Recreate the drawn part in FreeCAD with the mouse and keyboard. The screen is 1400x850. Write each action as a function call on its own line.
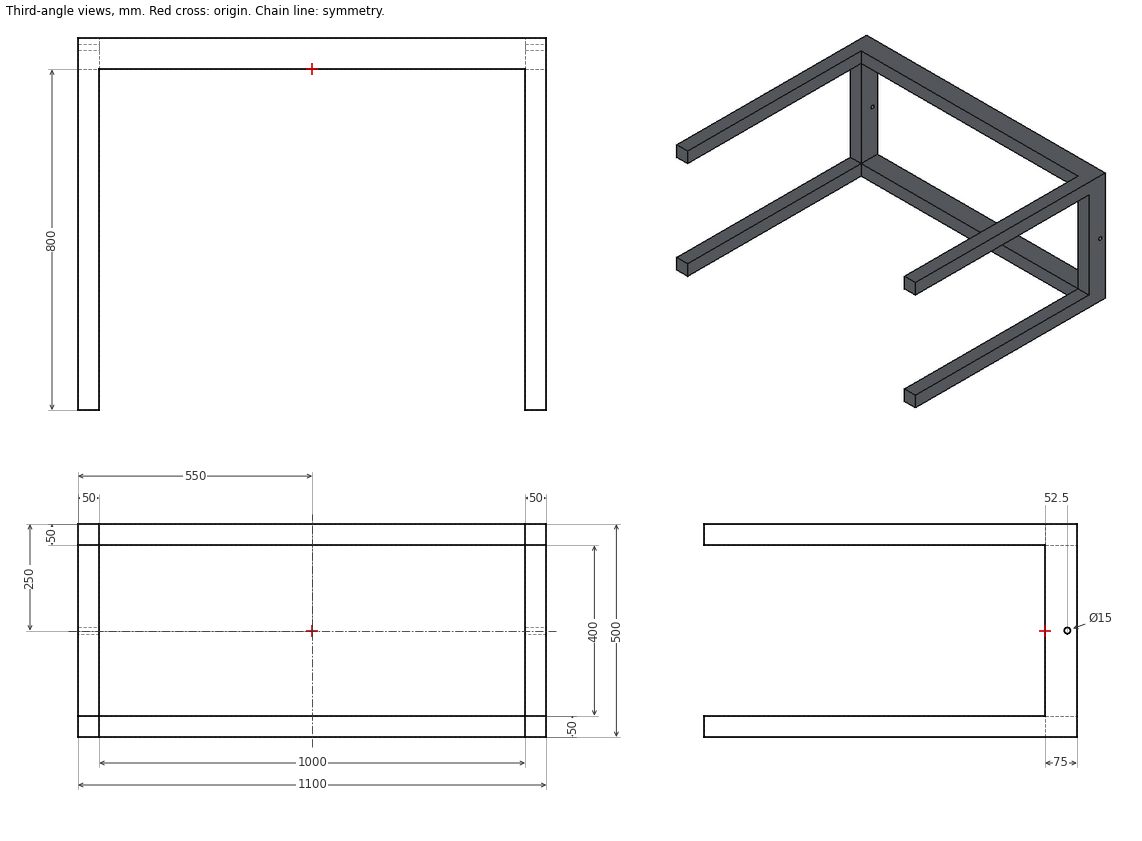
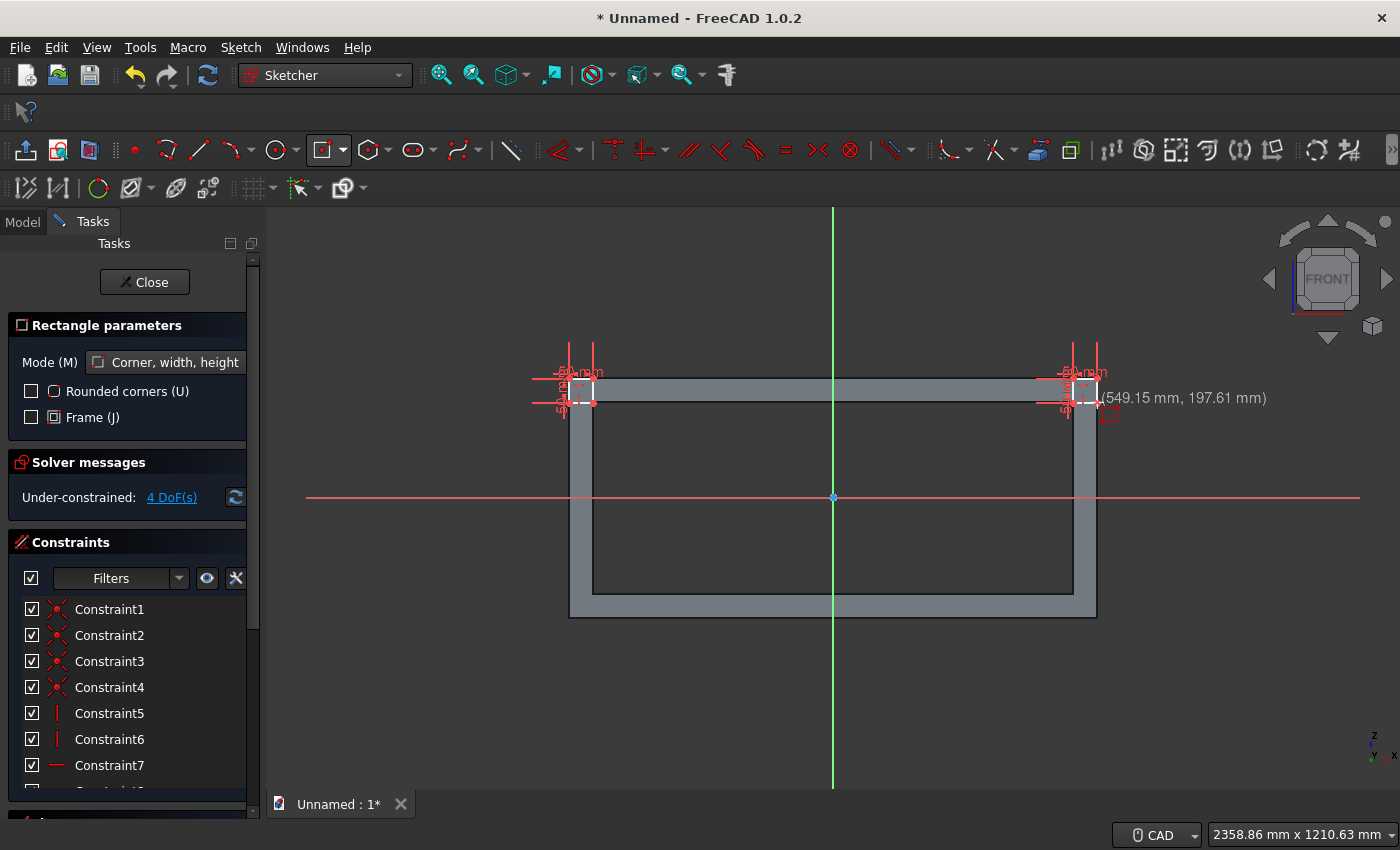
click(1073, 594)
move(1097, 618)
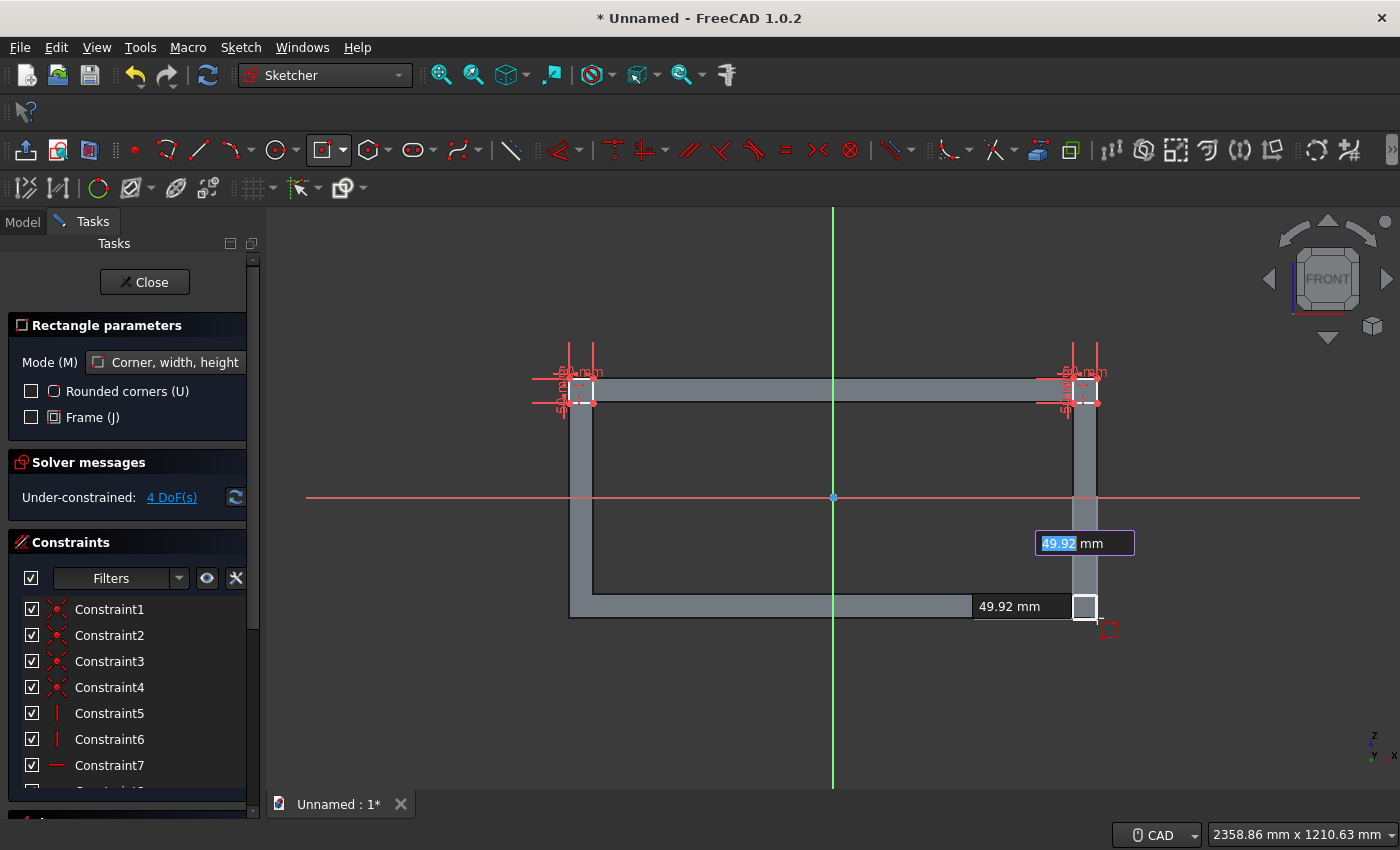
text(50)
key(Tab)
text(50)
key(Return)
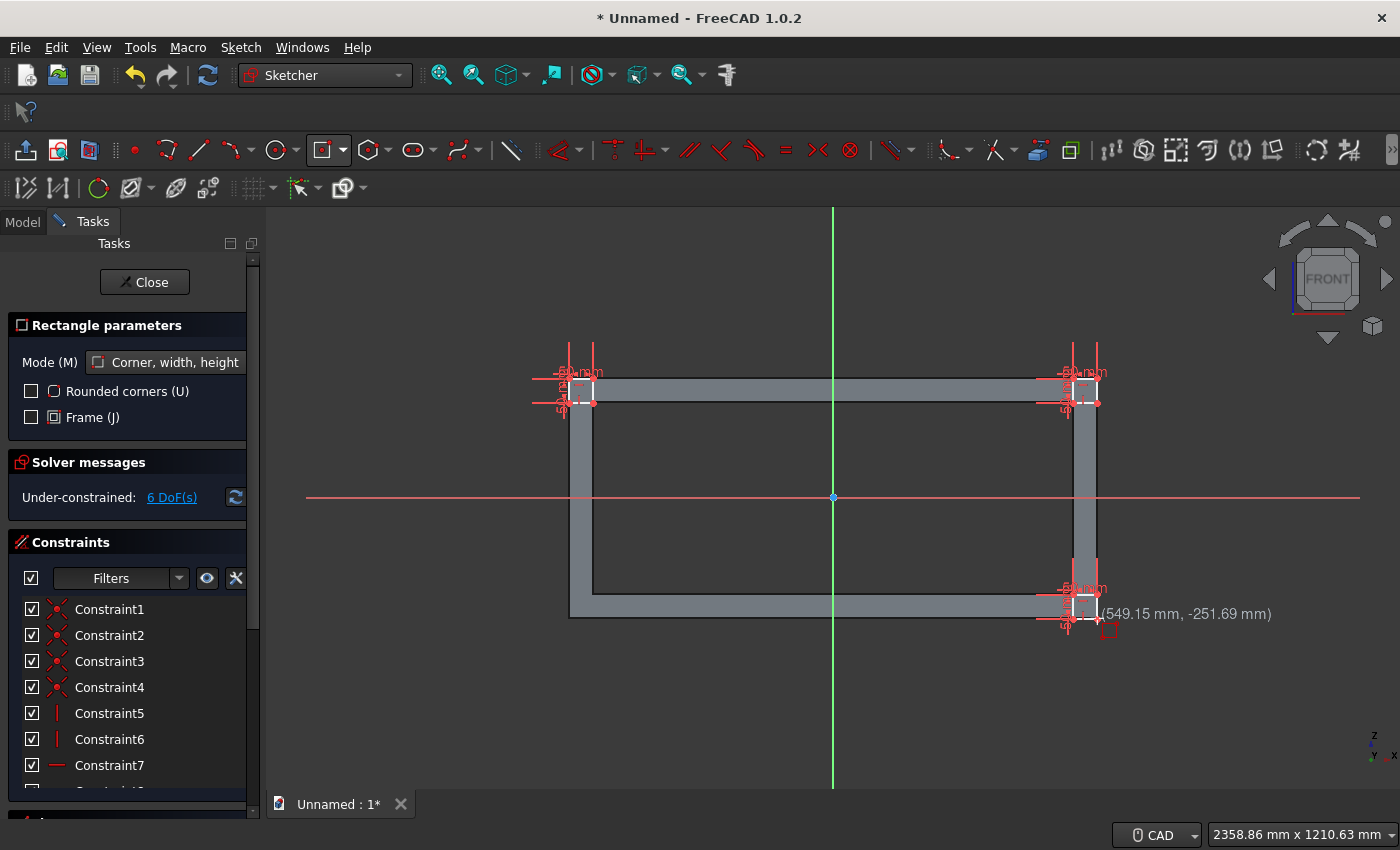
click(569, 594)
move(593, 618)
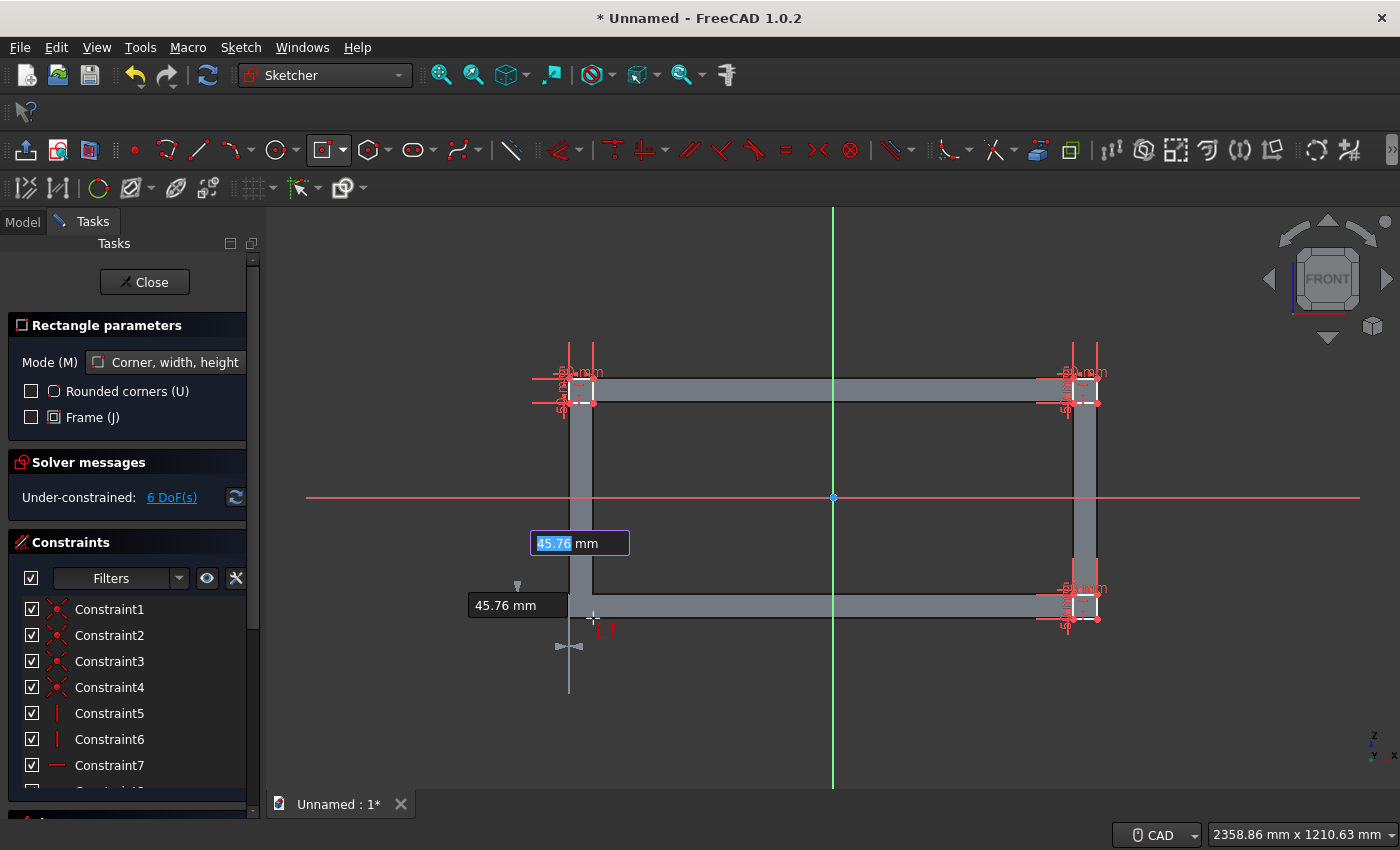
text(50)
key(Tab)
text(50)
key(Return)
key(Escape)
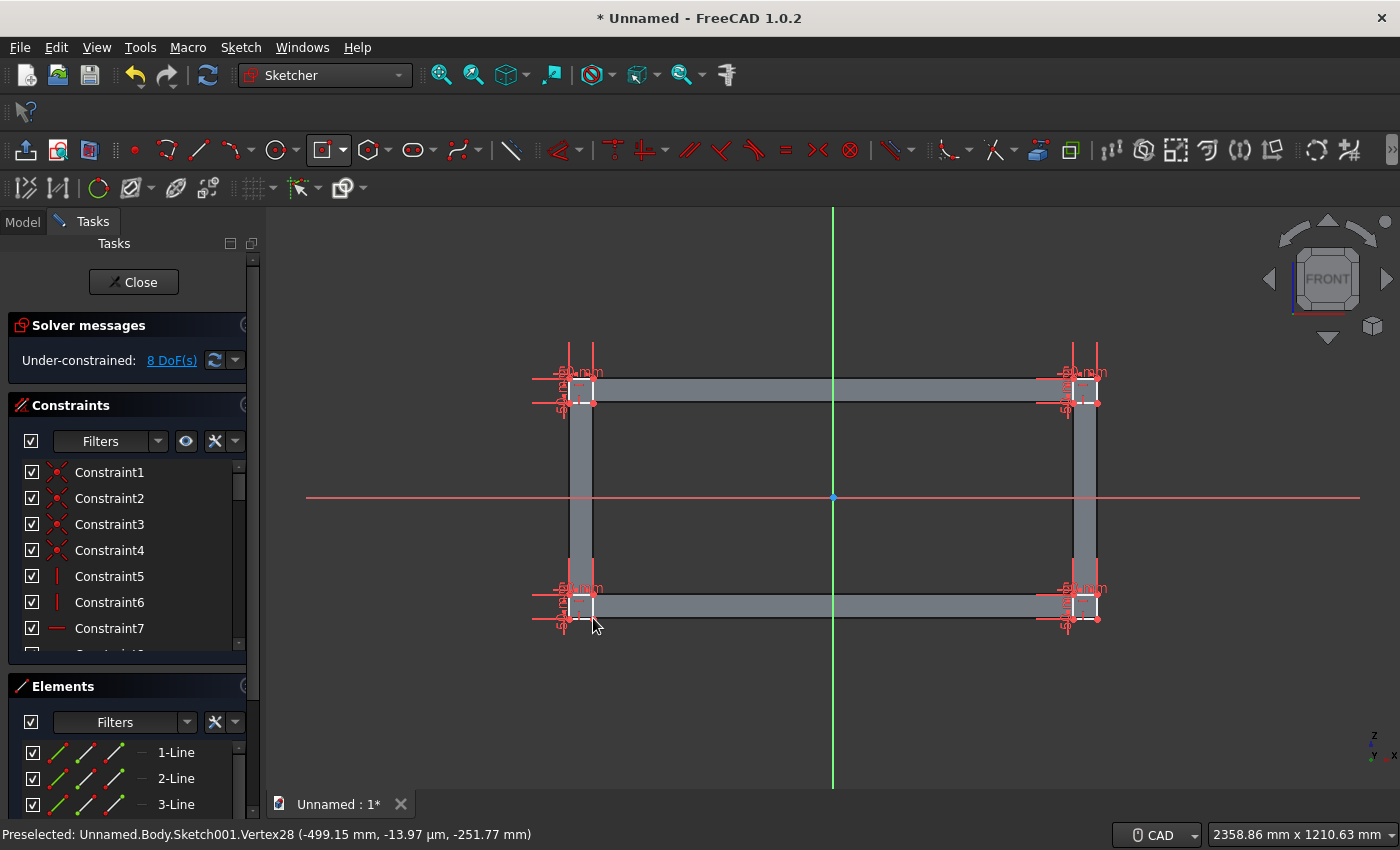
click(593, 379)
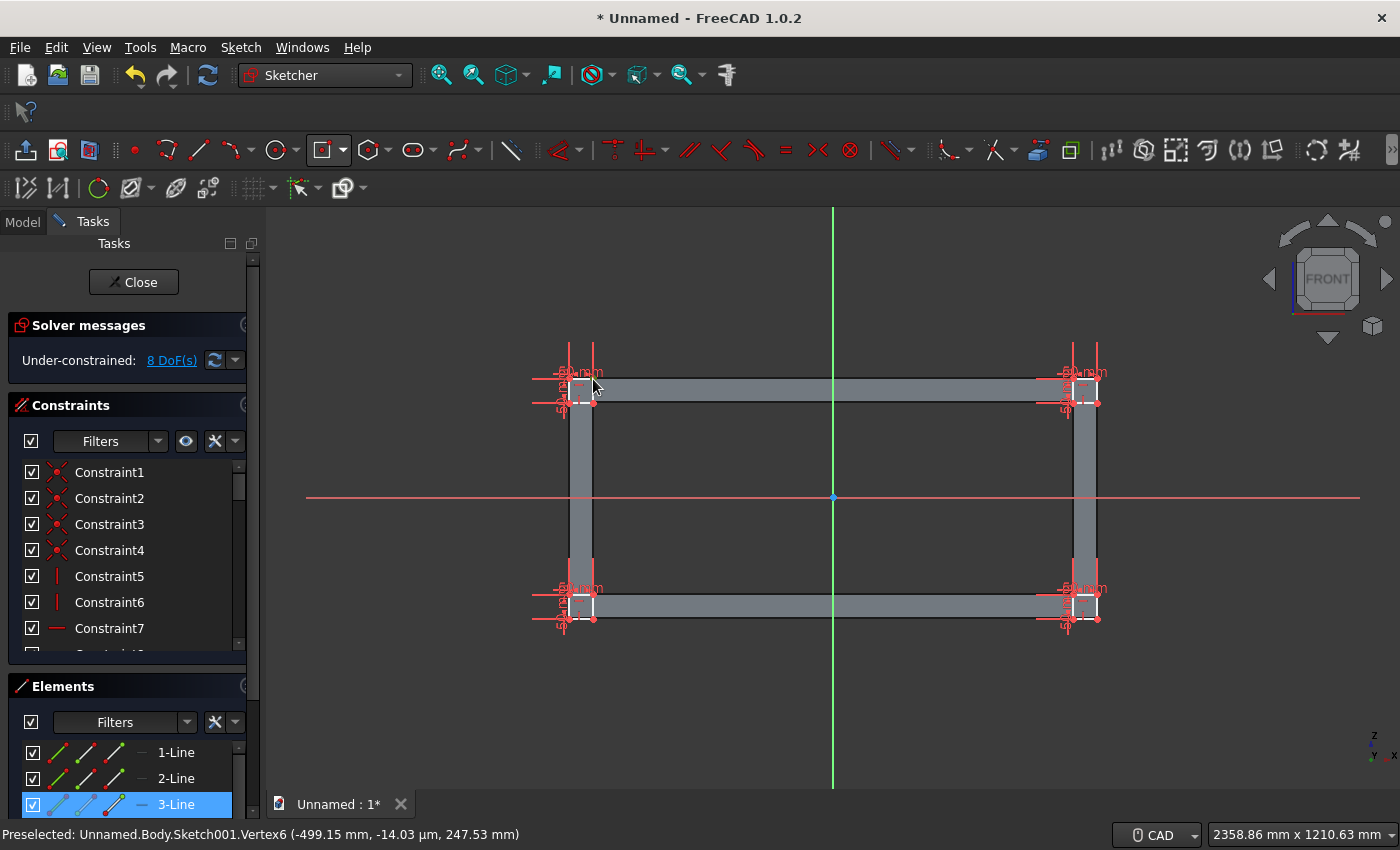
click(1073, 379)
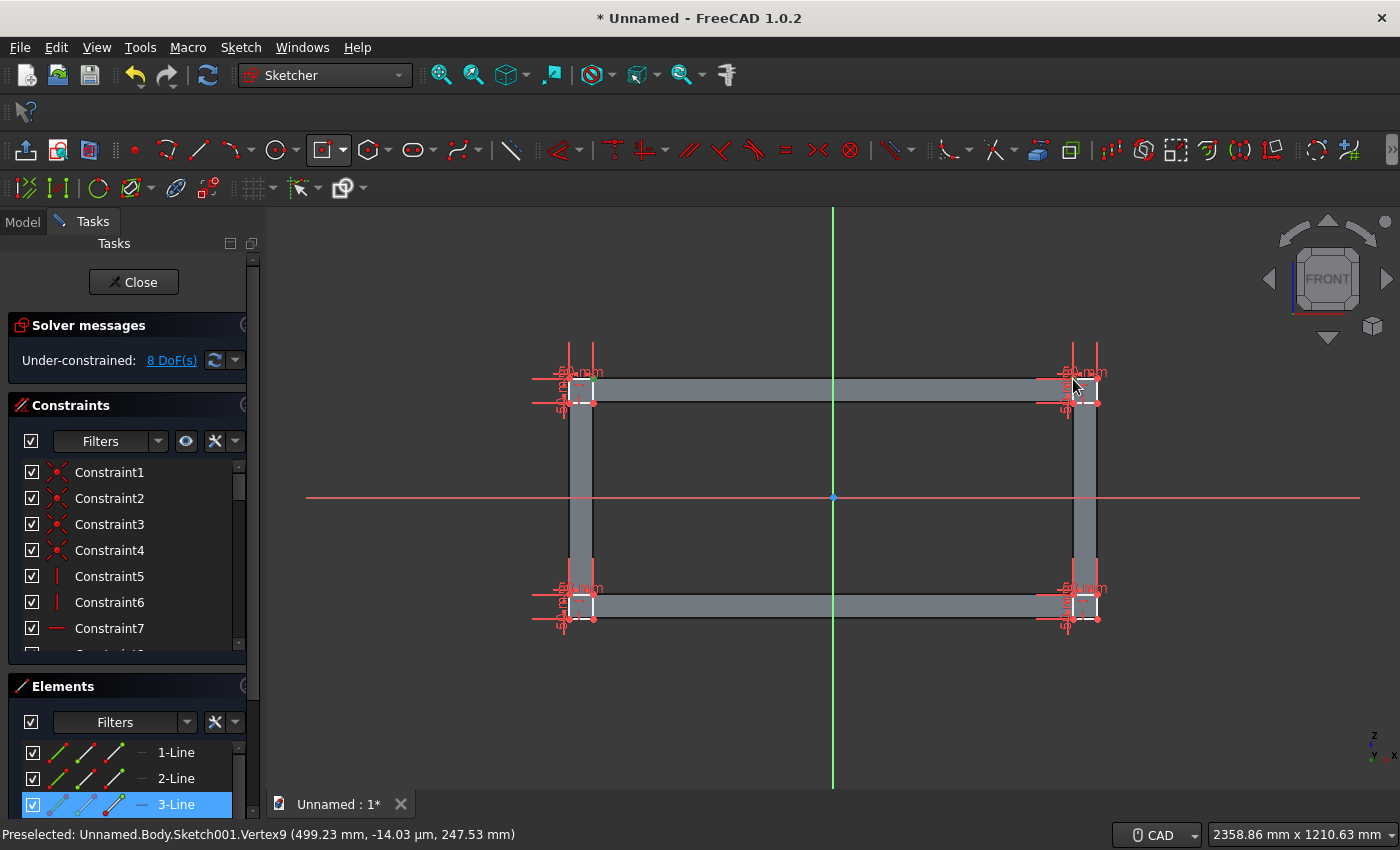
click(833, 723)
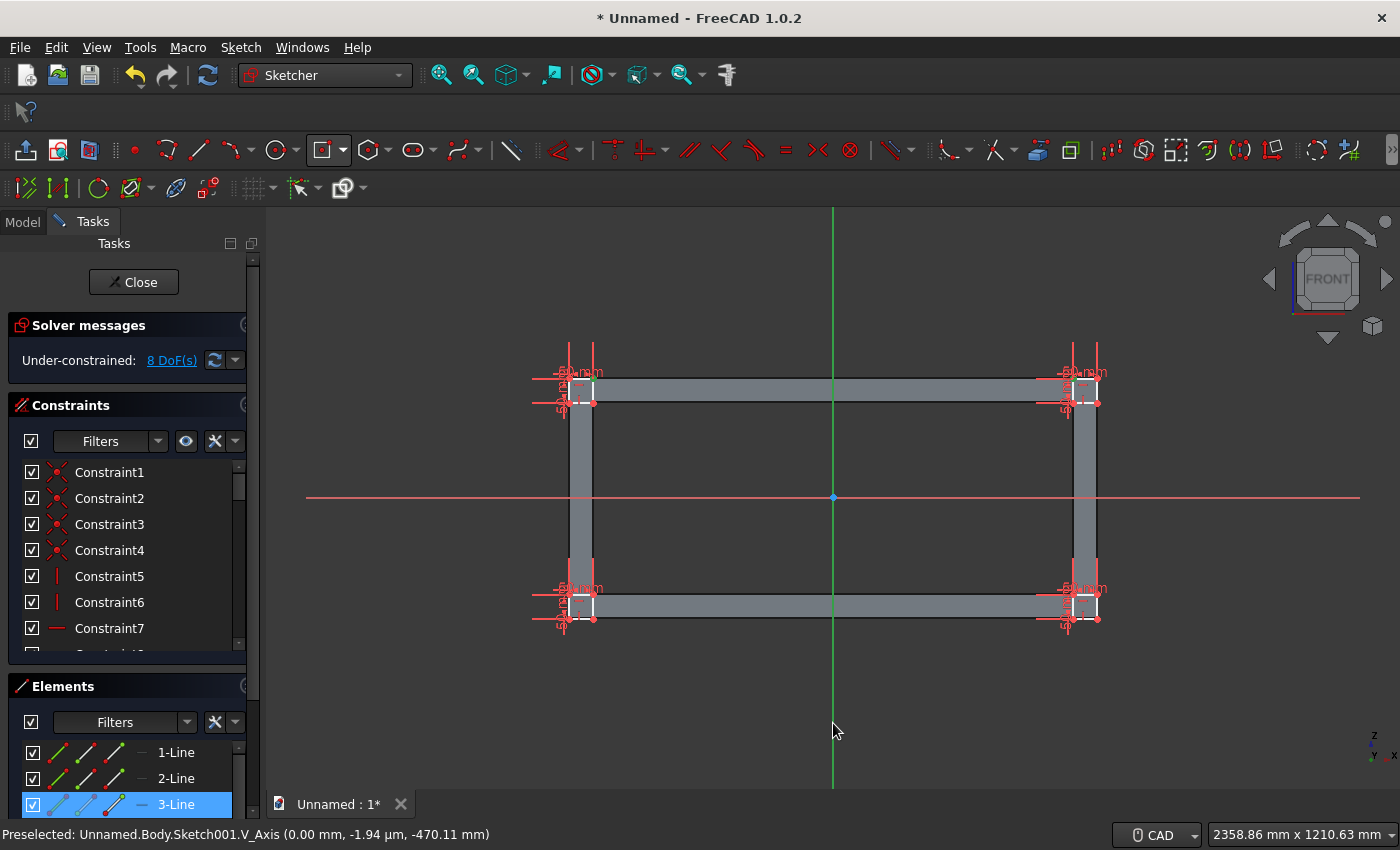
click(818, 150)